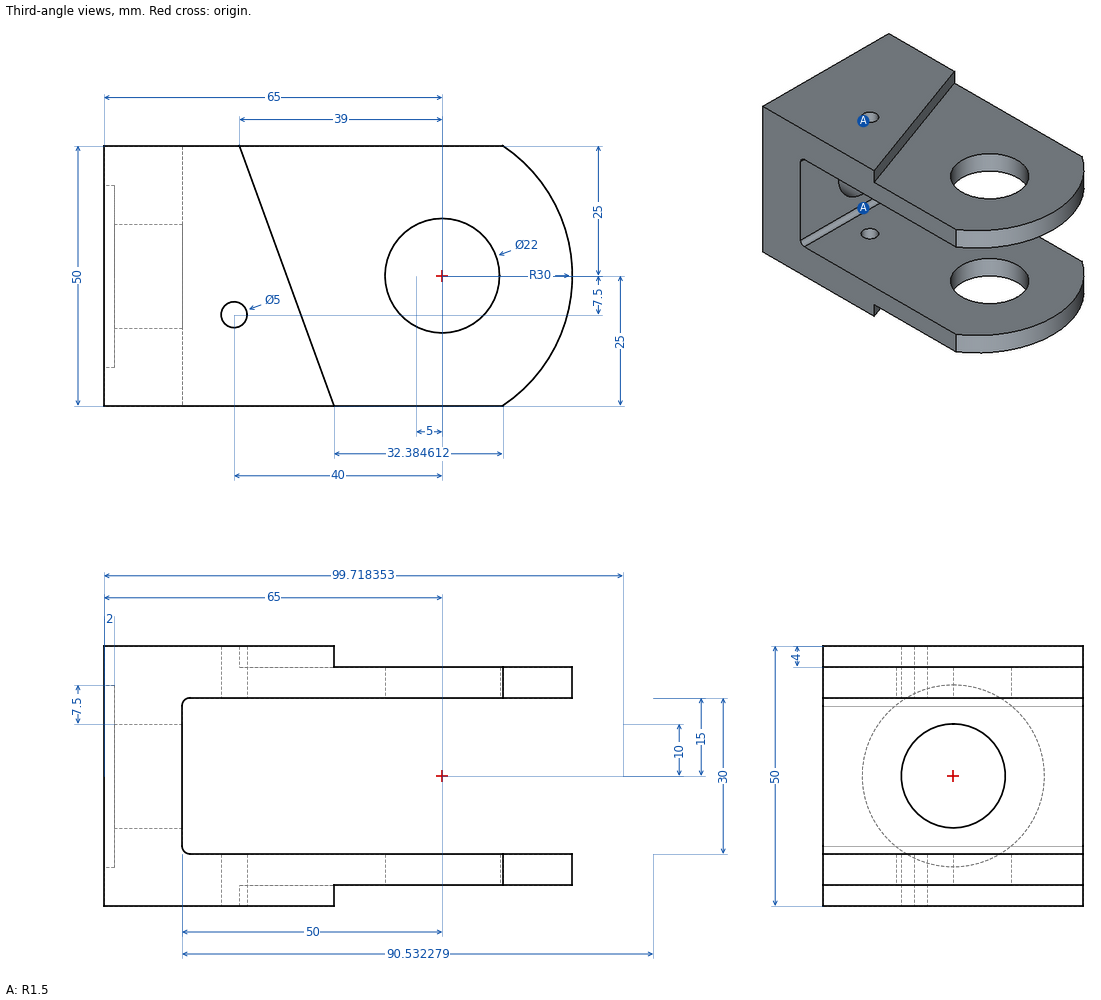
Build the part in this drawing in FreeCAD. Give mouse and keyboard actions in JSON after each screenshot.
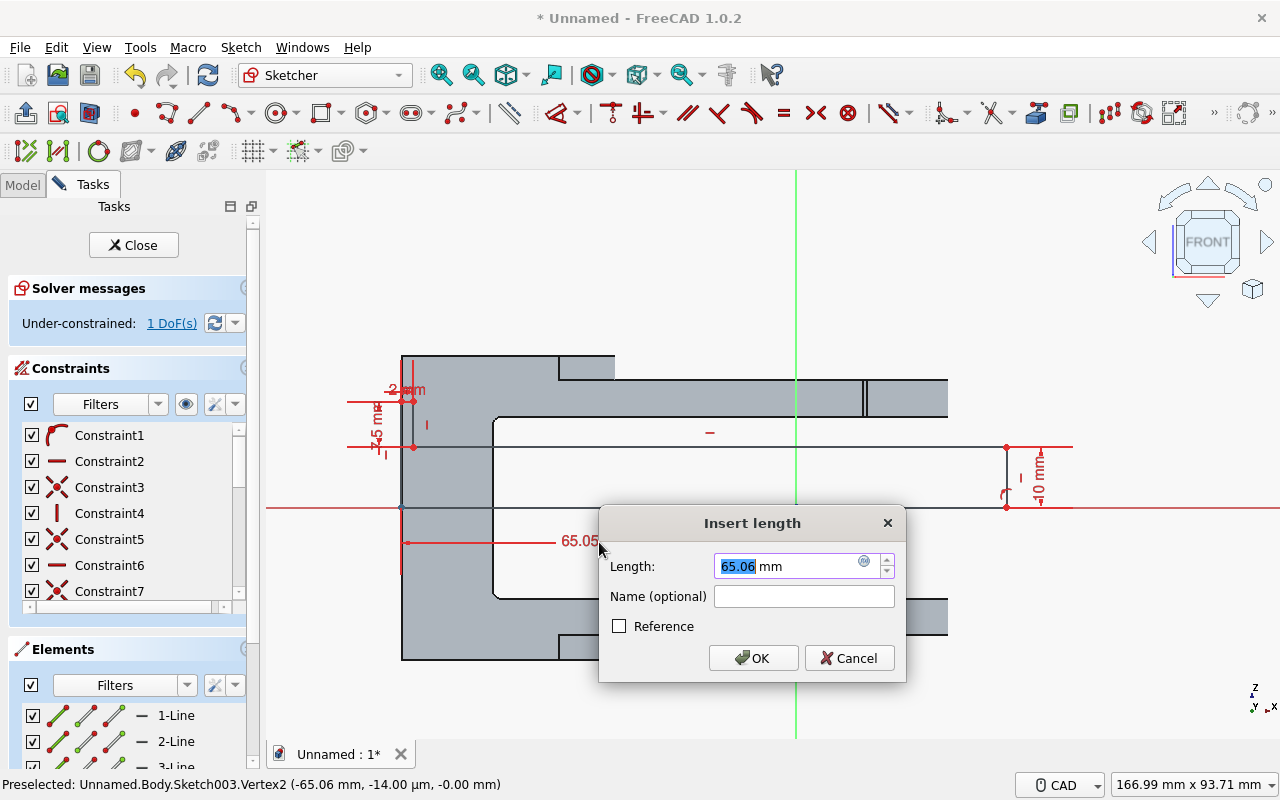
{"action": "type", "text": "65"}
{"action": "key", "text": "Return"}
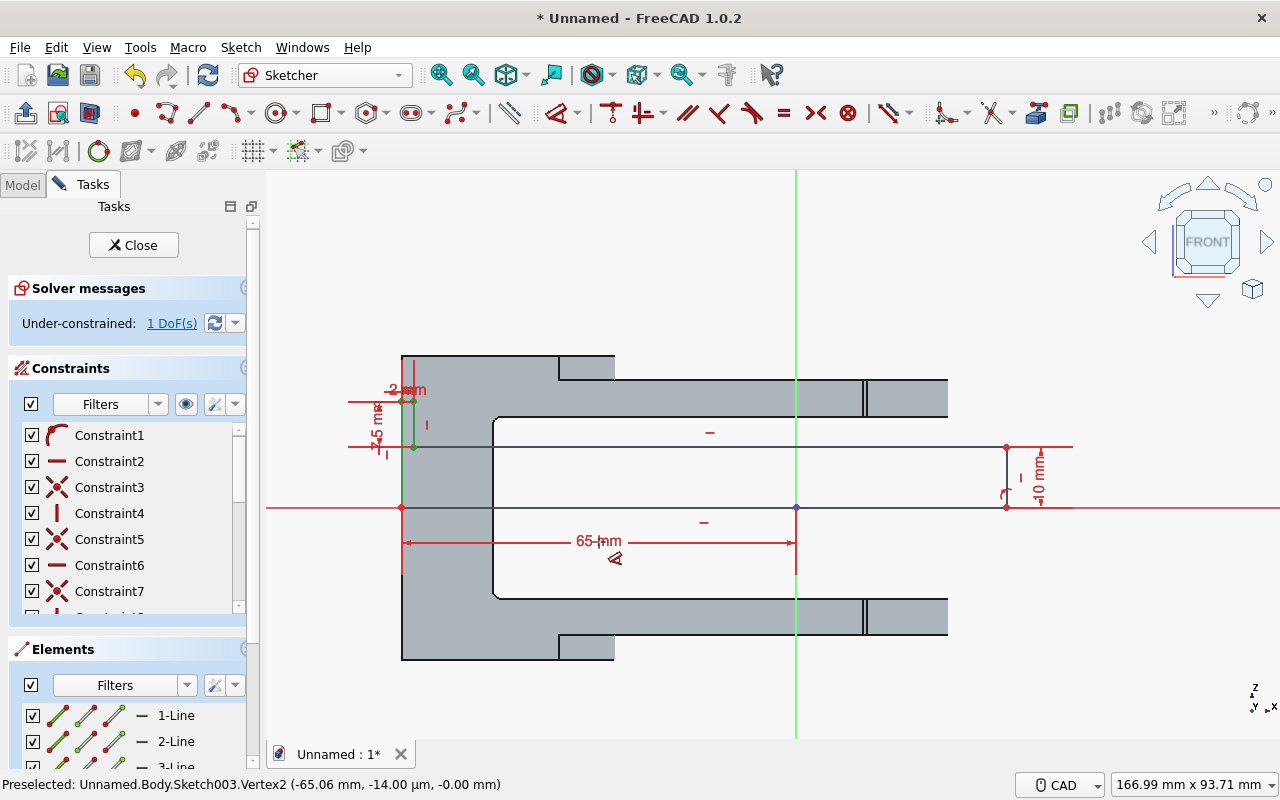
{"action": "left_click", "coordinate": [825, 508]}
{"action": "left_click", "coordinate": [704, 542]}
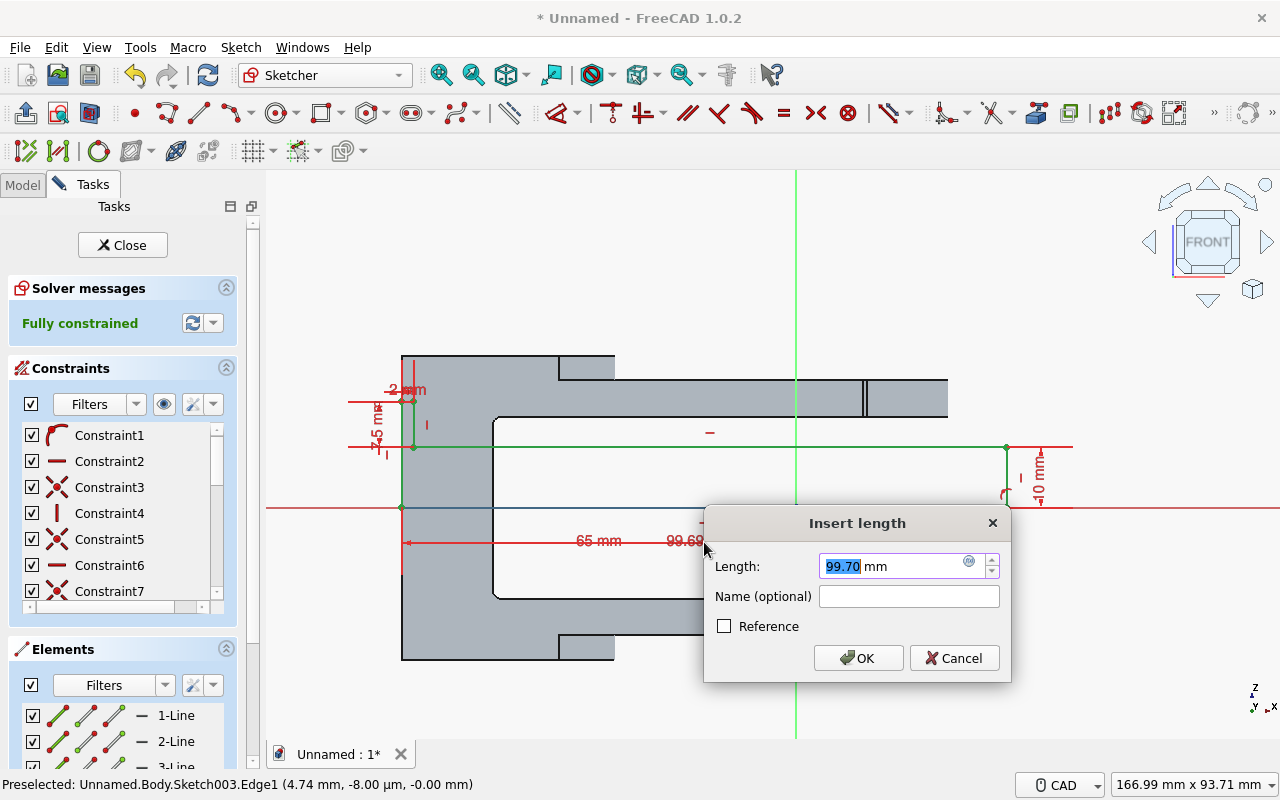
{"action": "type", "text": "99.718353"}
{"action": "key", "text": "Return"}
{"action": "key", "text": "Escape"}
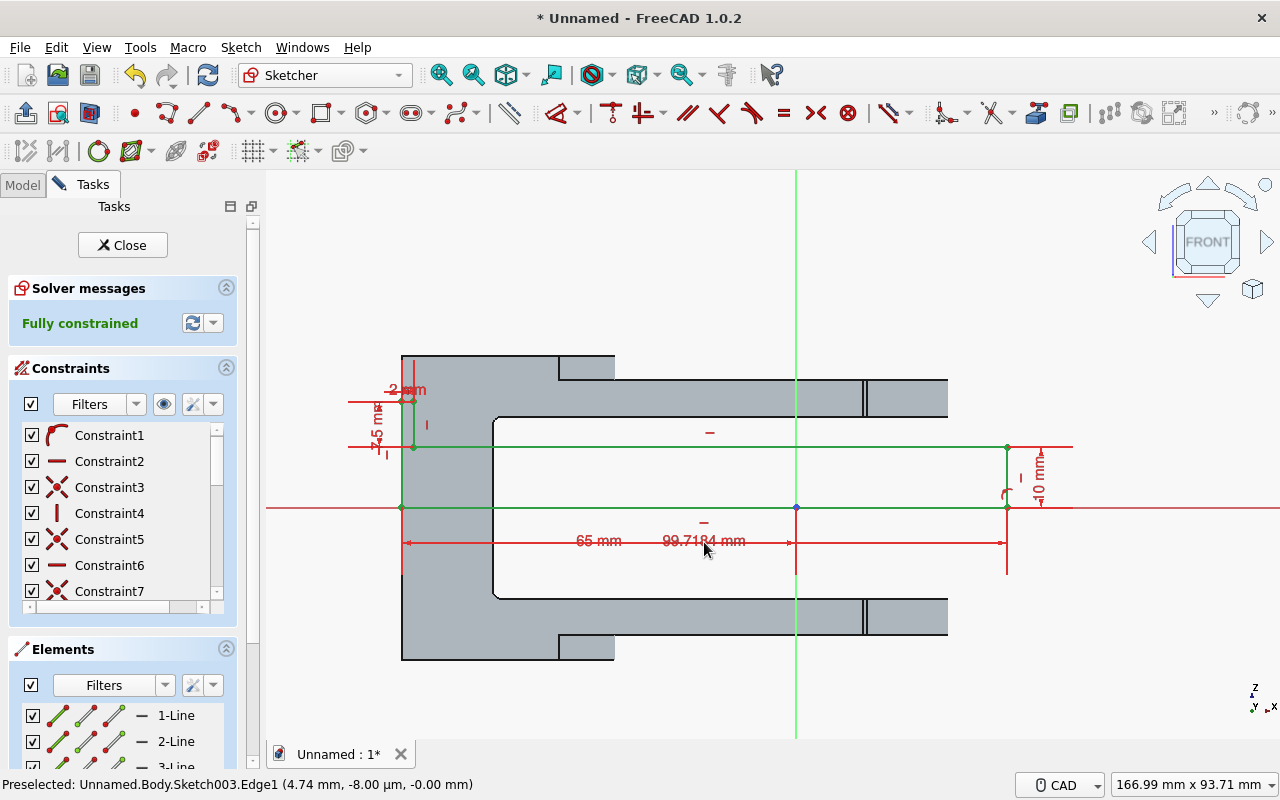
{"action": "left_click", "coordinate": [123, 245]}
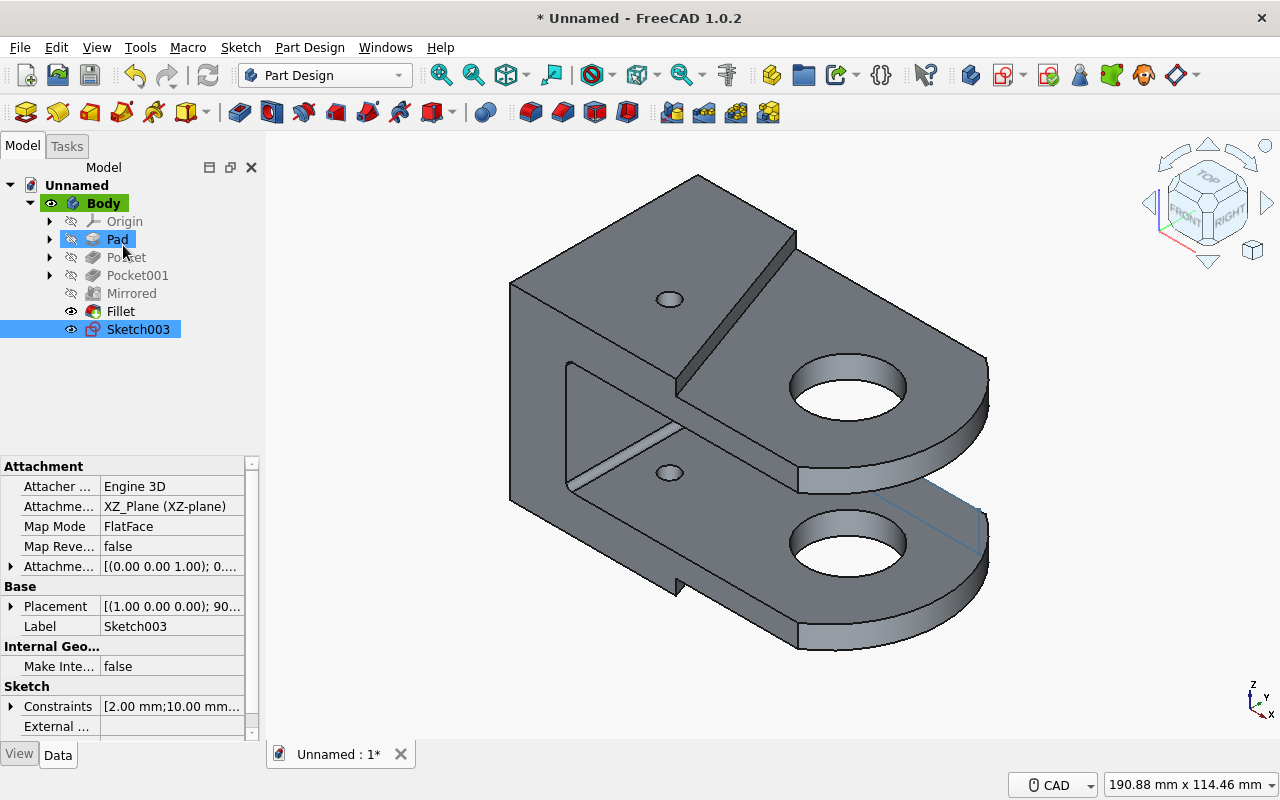
{"action": "left_click", "coordinate": [304, 112]}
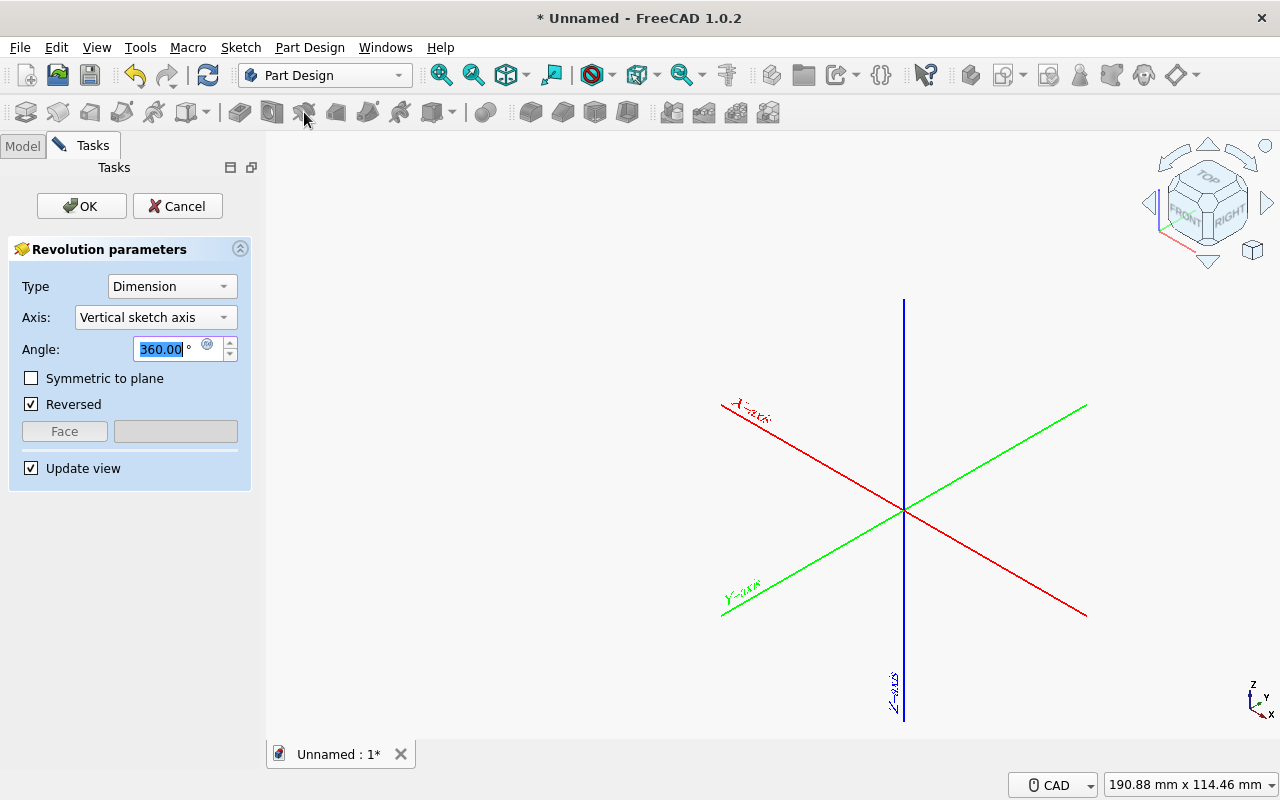
{"action": "left_click", "coordinate": [156, 318]}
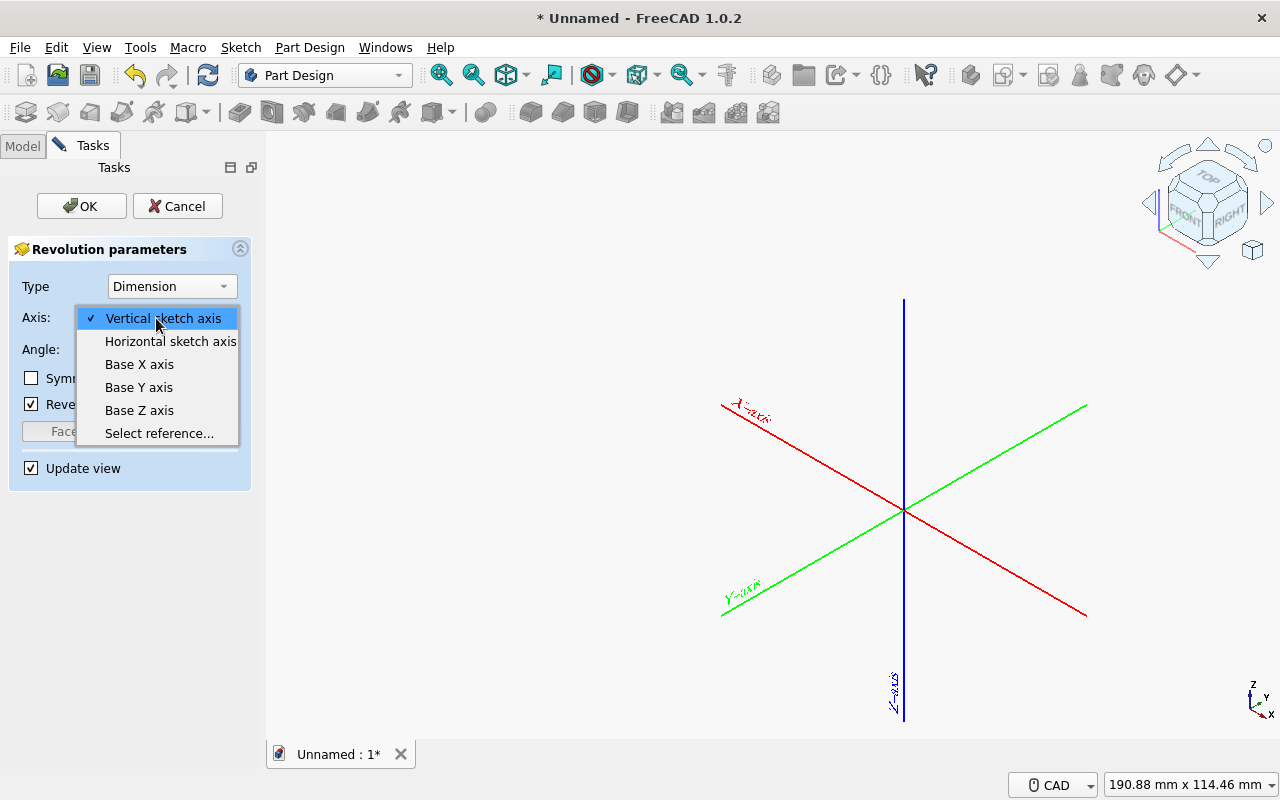
{"action": "left_click", "coordinate": [156, 342]}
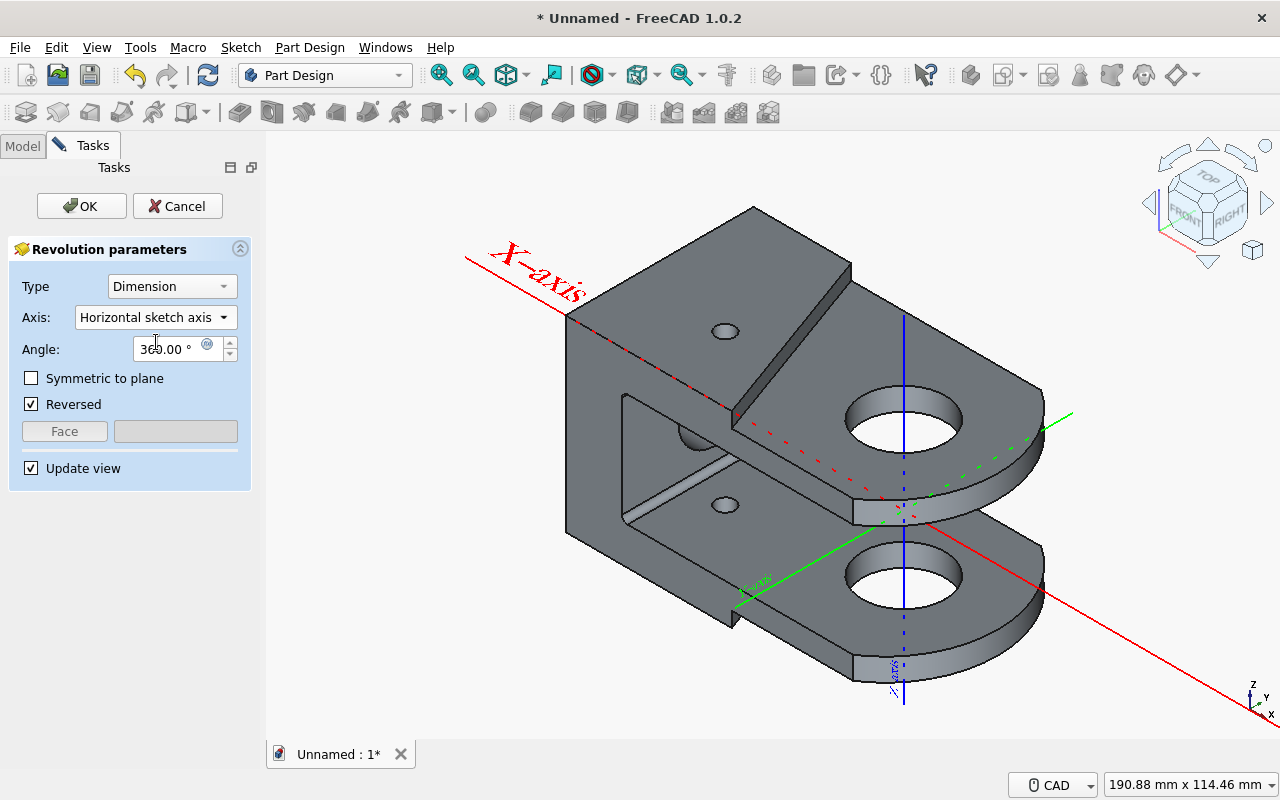
{"action": "left_click", "coordinate": [82, 206]}